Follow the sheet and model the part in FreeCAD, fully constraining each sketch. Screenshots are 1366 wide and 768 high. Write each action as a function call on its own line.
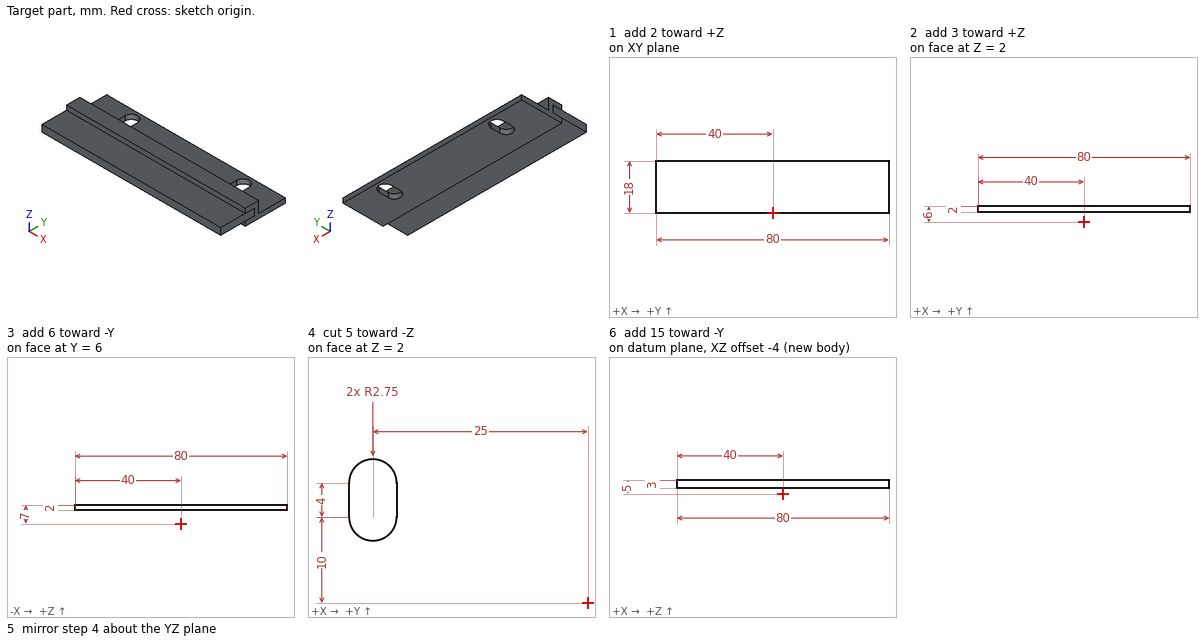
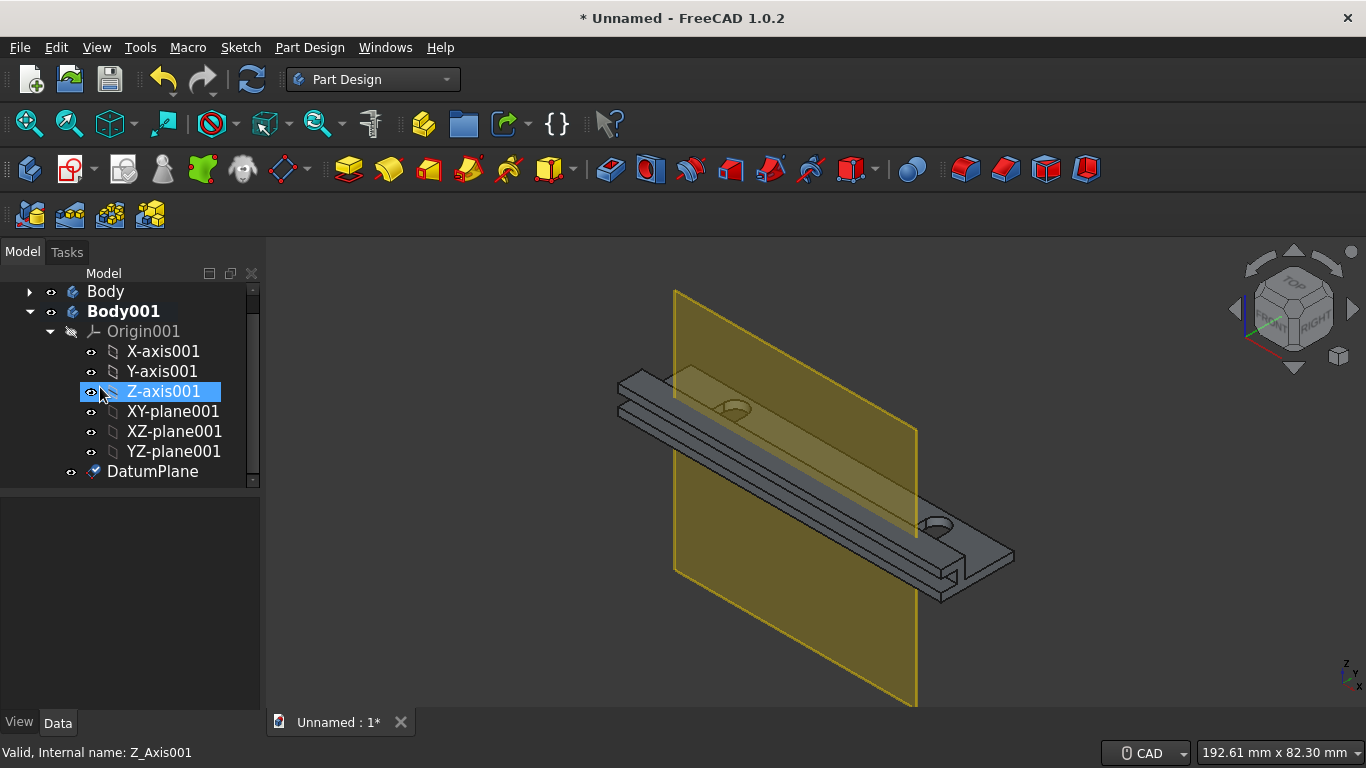
click(116, 472)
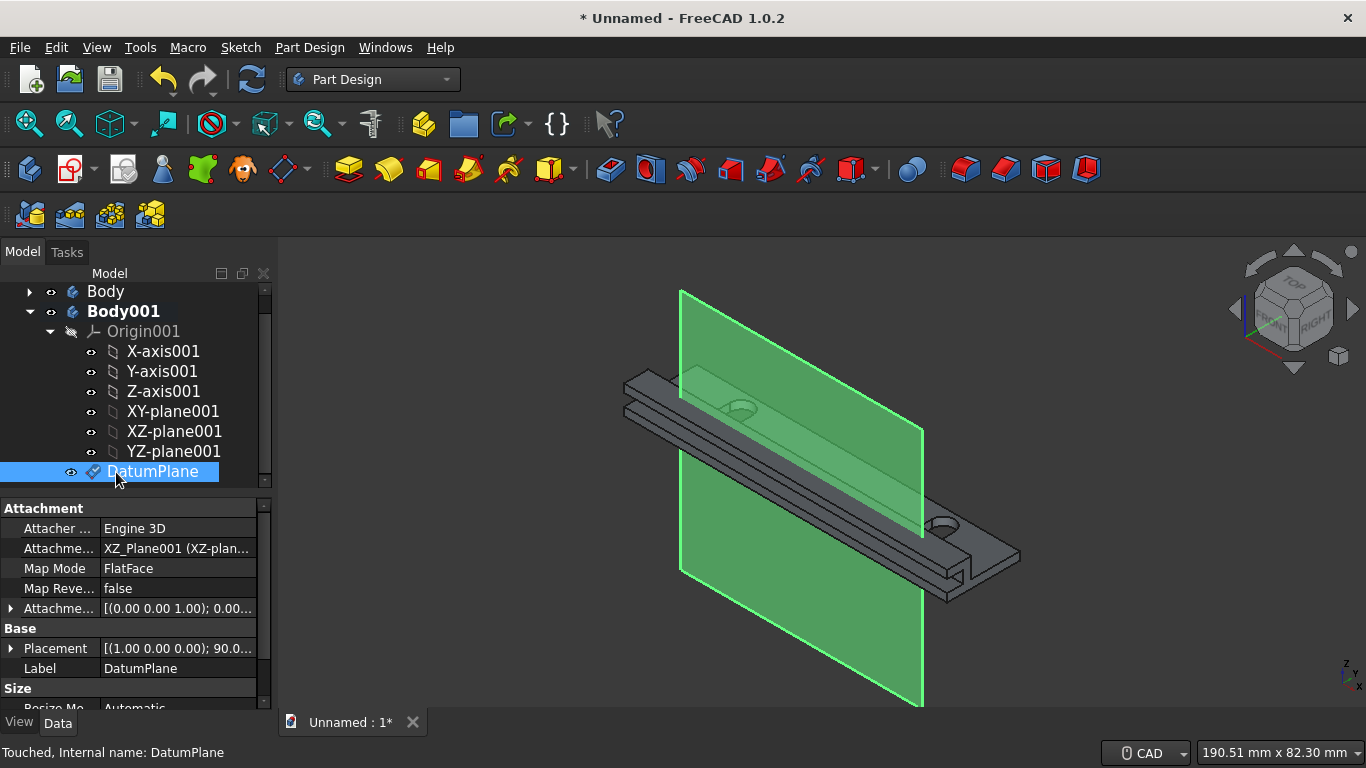
click(70, 170)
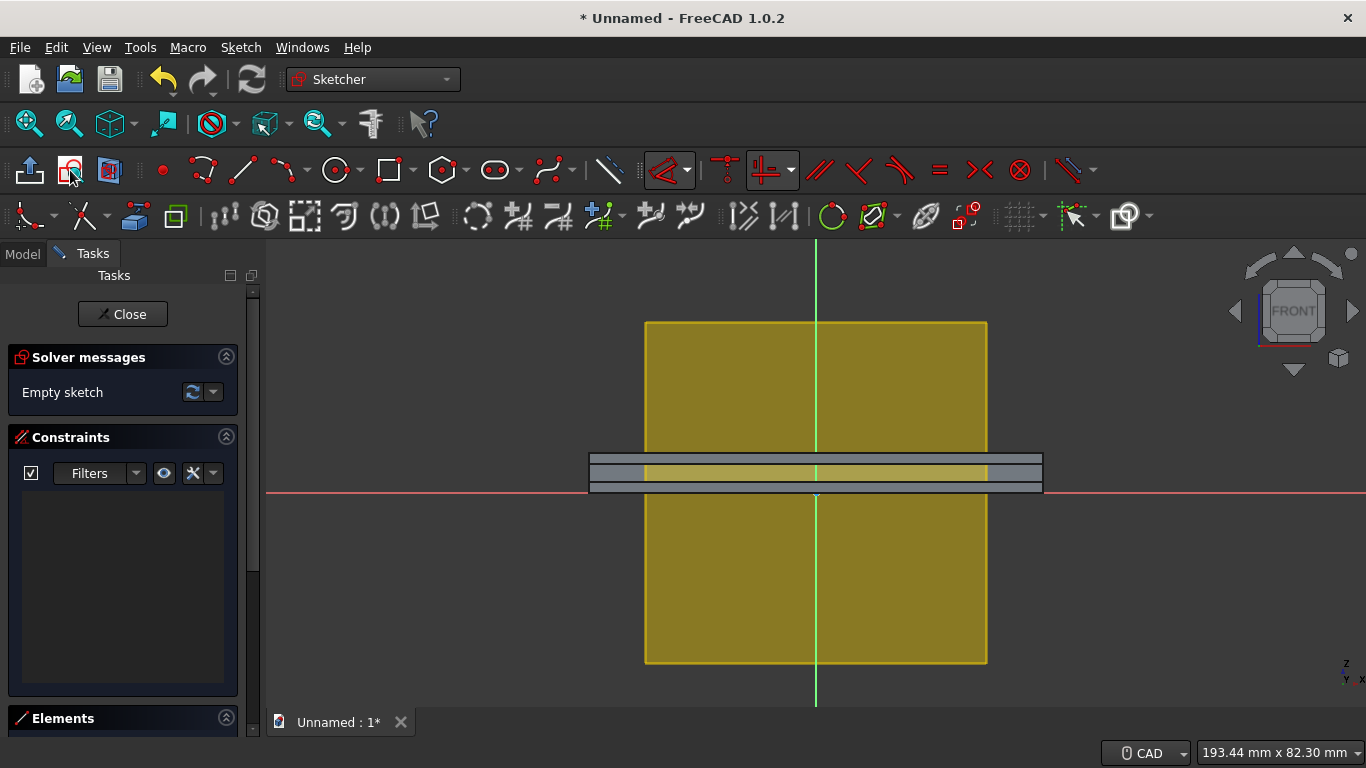
scroll(955, 490, up, 2)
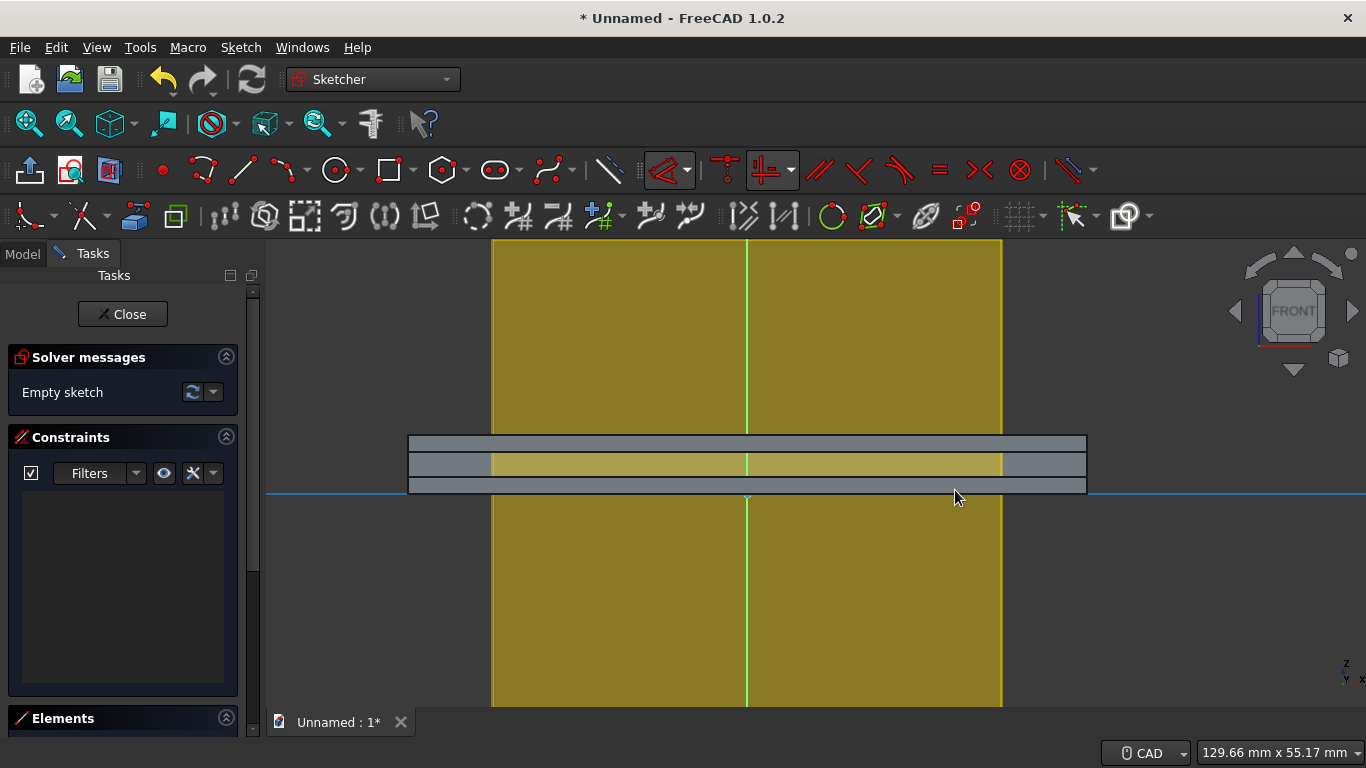
click(390, 170)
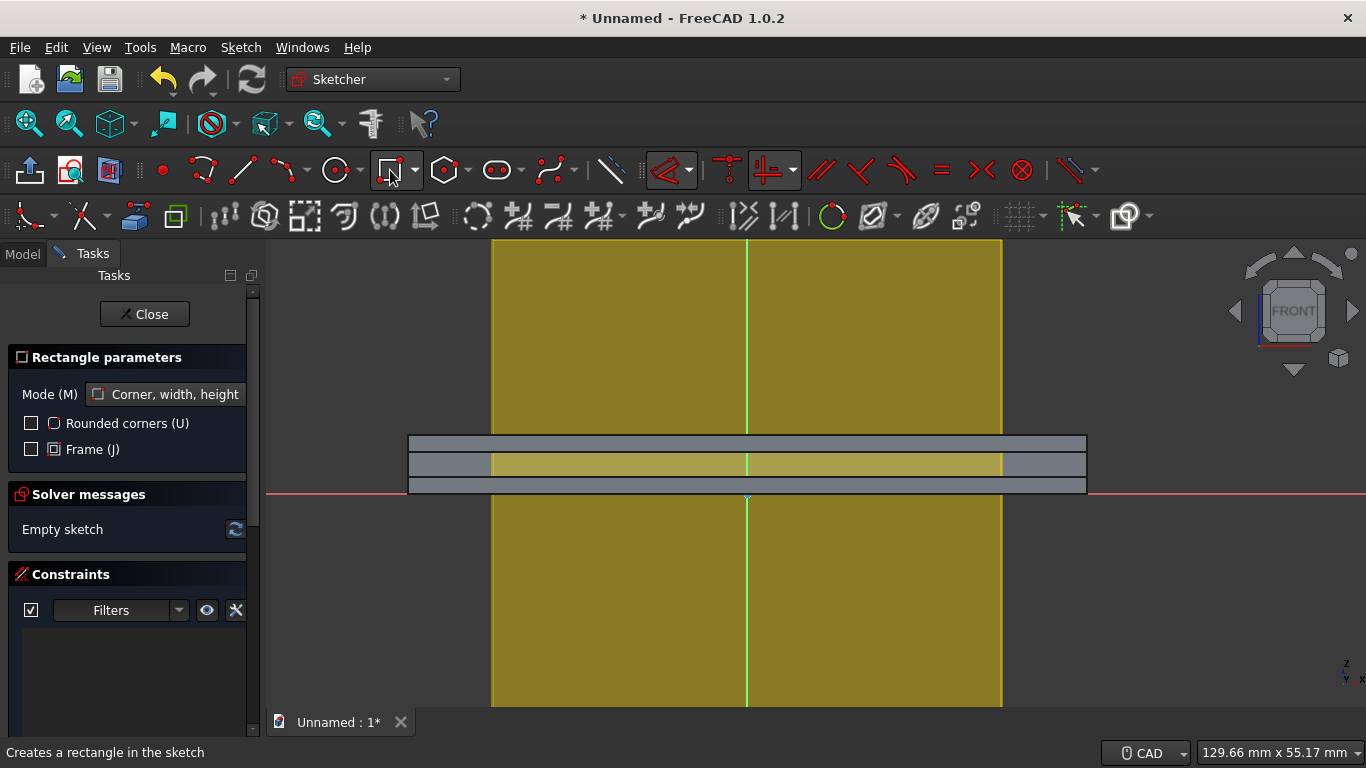
click(408, 452)
click(1087, 477)
key(Escape)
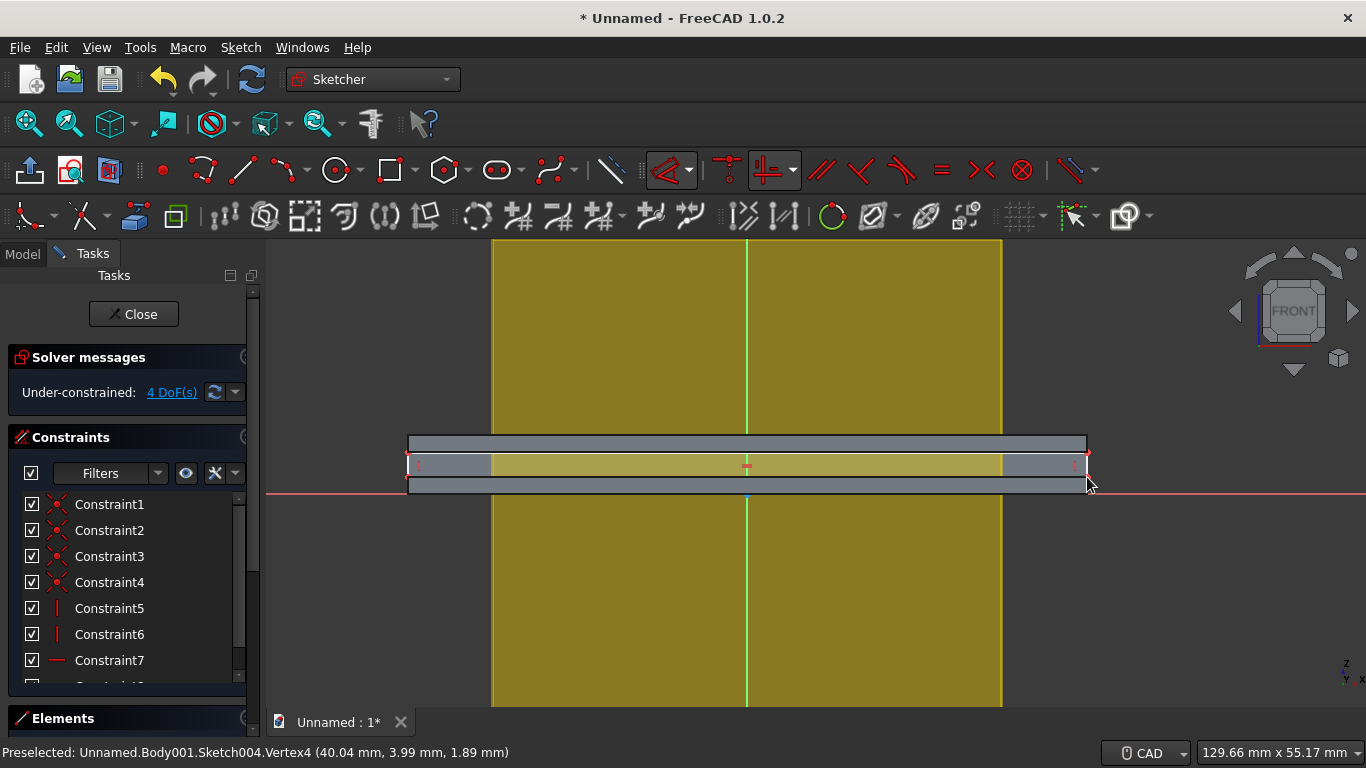
scroll(408, 463, up, 3)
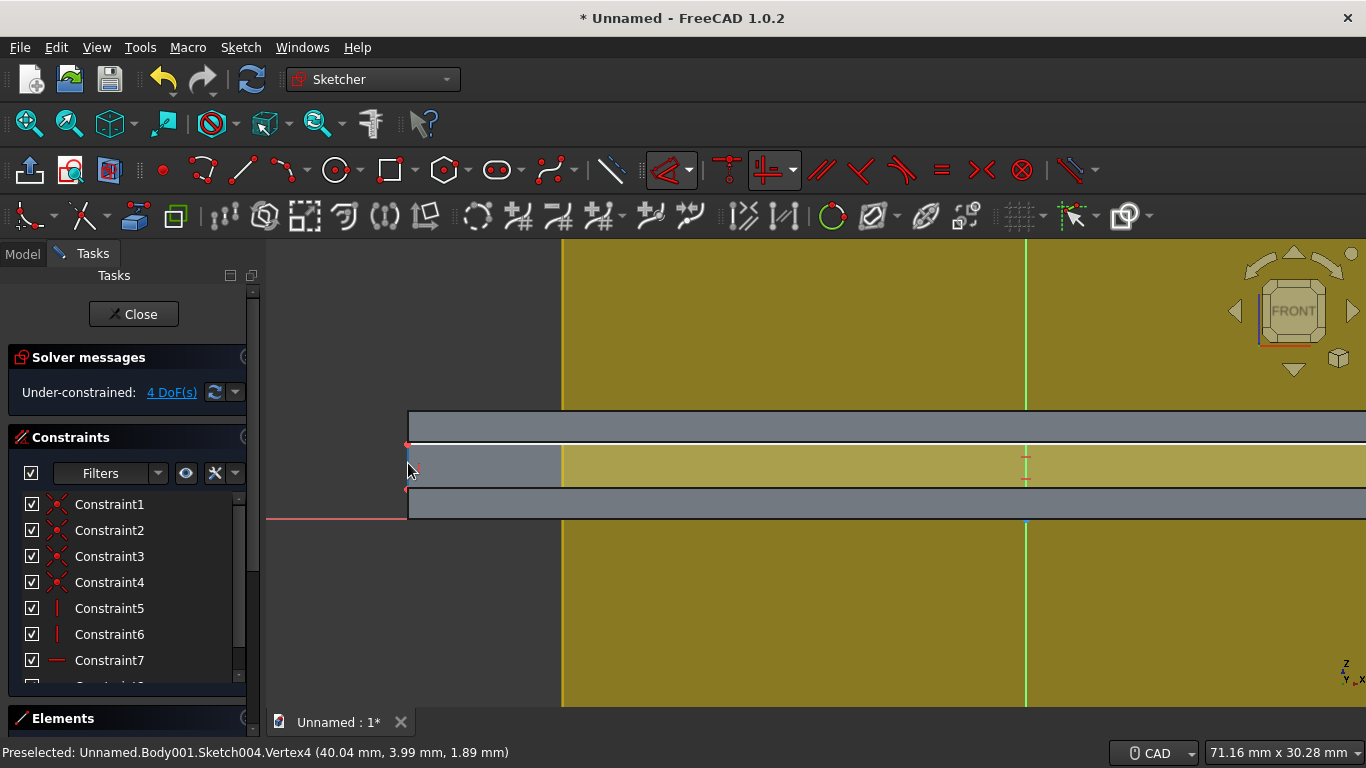
click(408, 463)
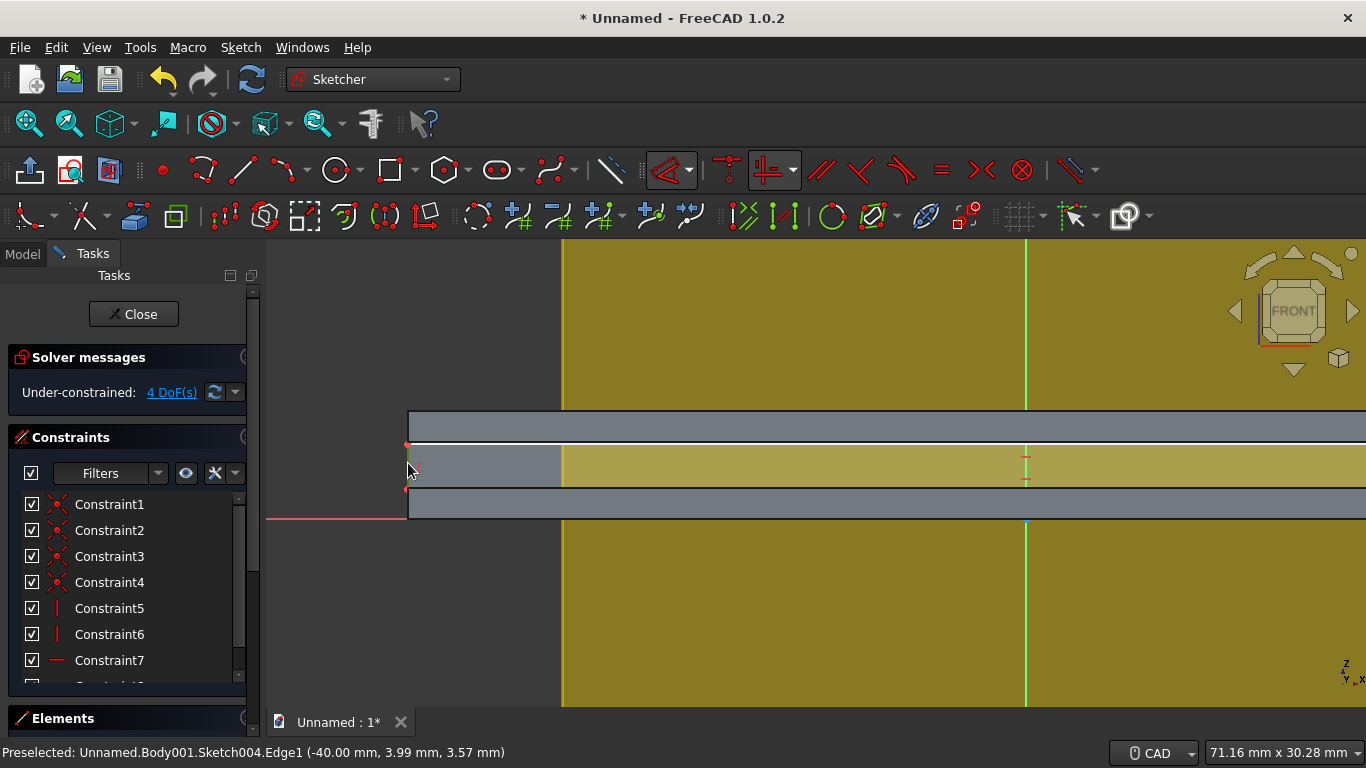
key(i)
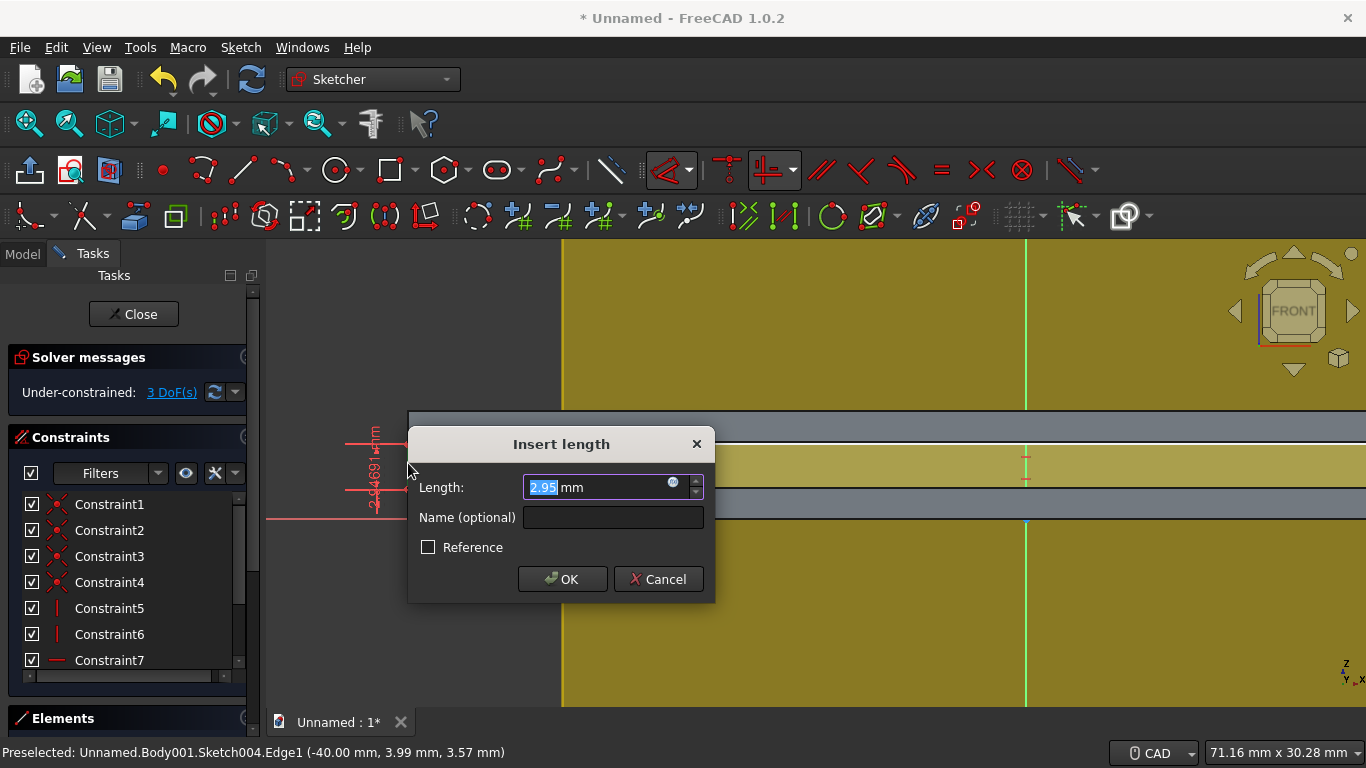
text(3)
key(Return)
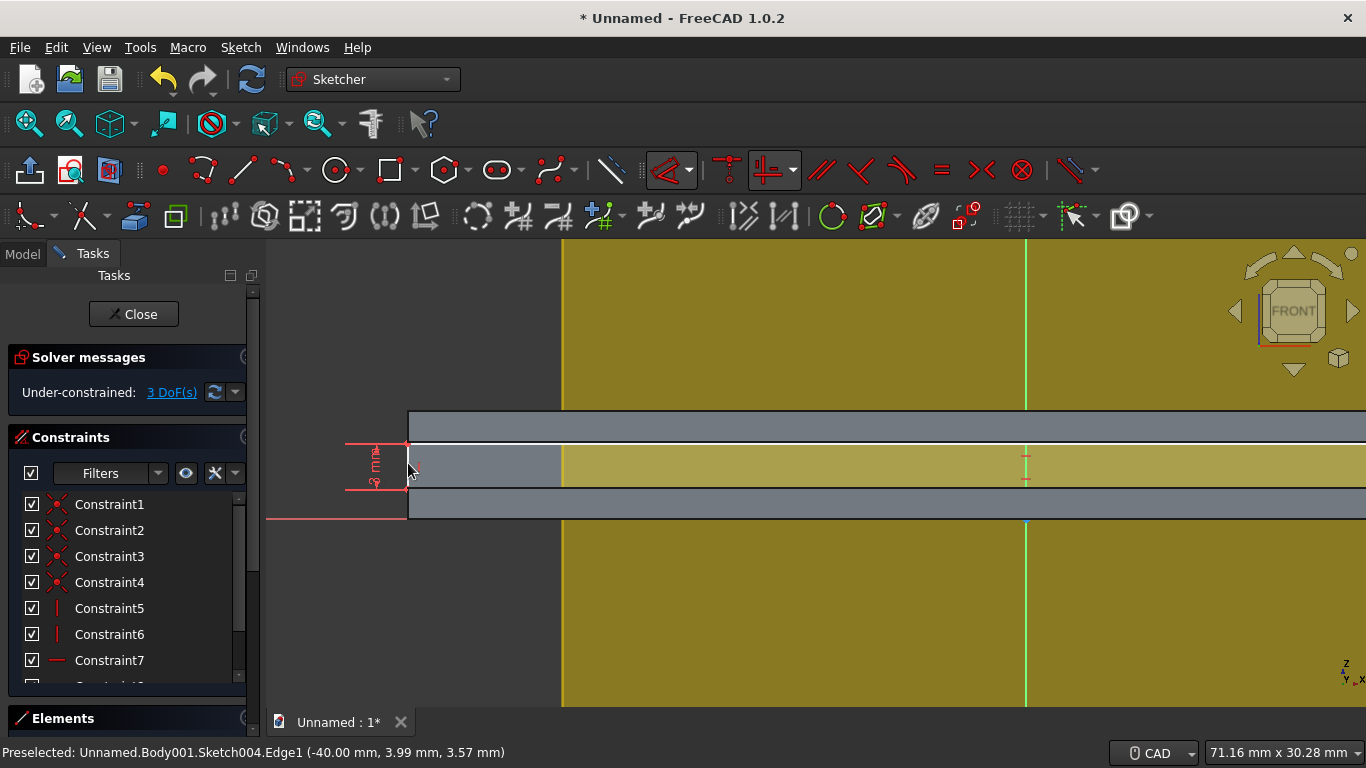
click(779, 490)